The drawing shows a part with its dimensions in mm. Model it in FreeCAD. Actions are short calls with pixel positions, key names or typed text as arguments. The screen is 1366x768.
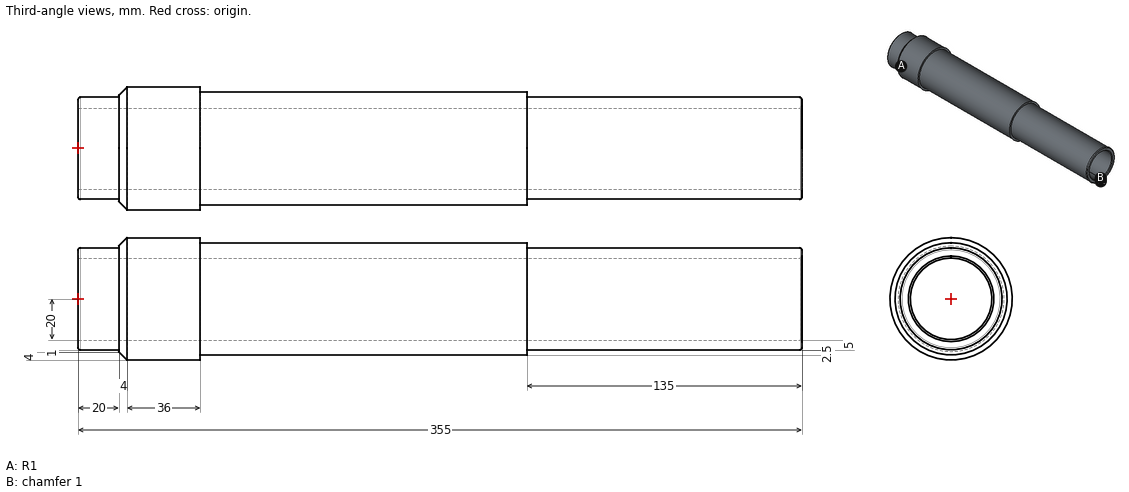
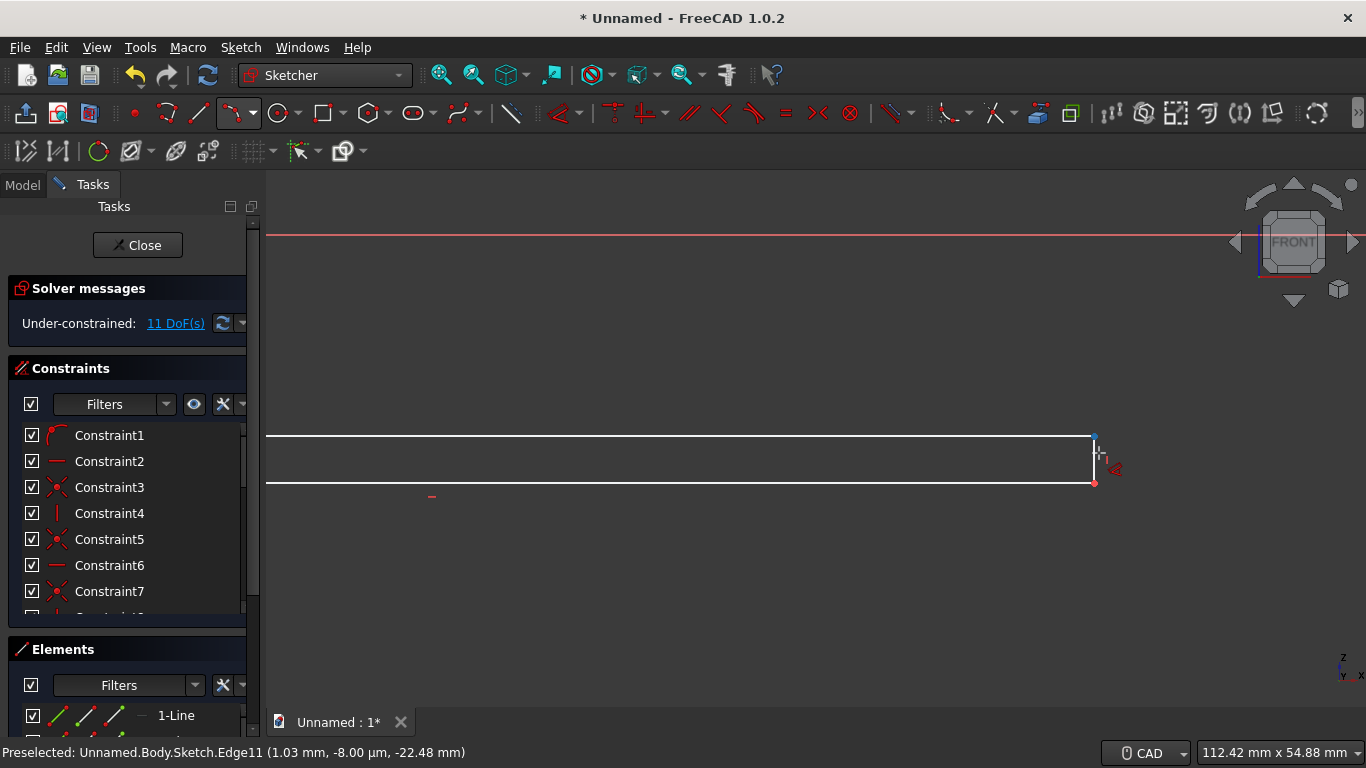
click(1094, 450)
click(1128, 460)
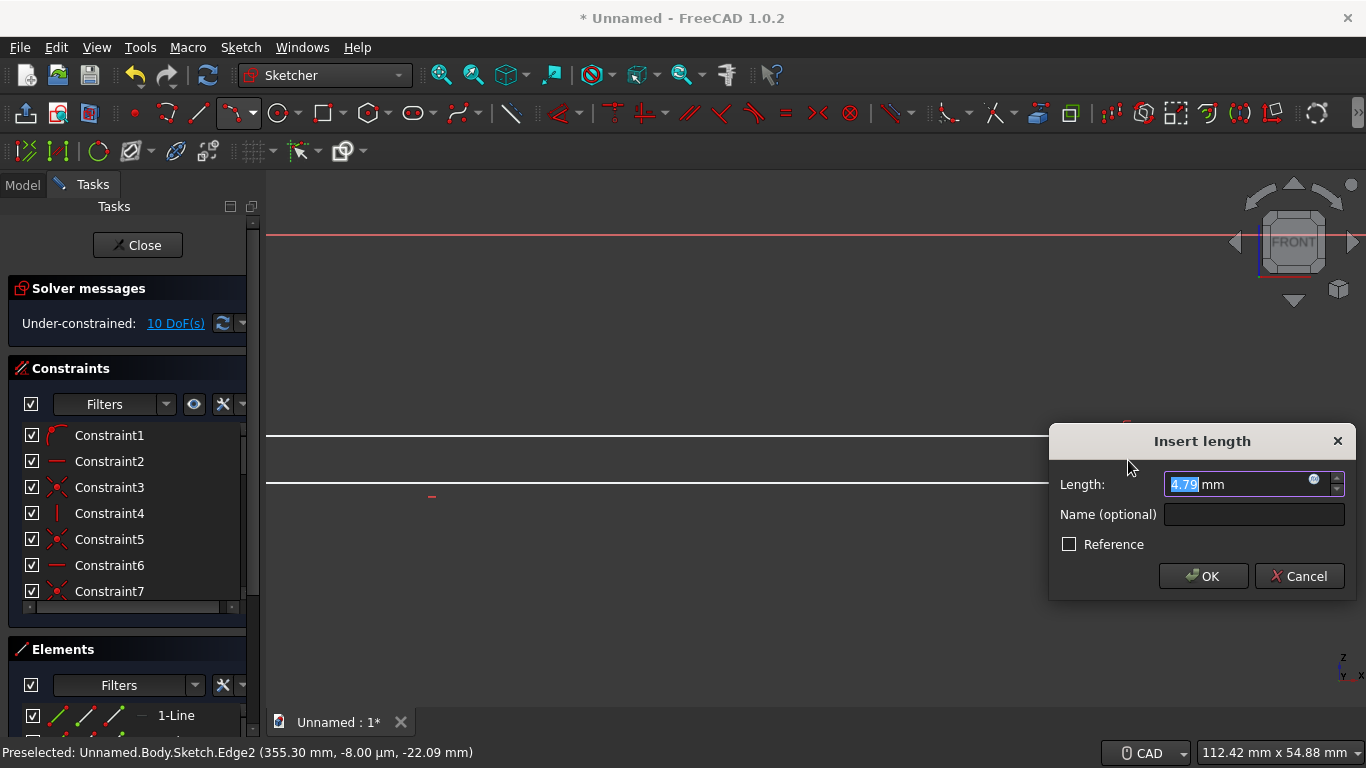
text(5)
key(Return)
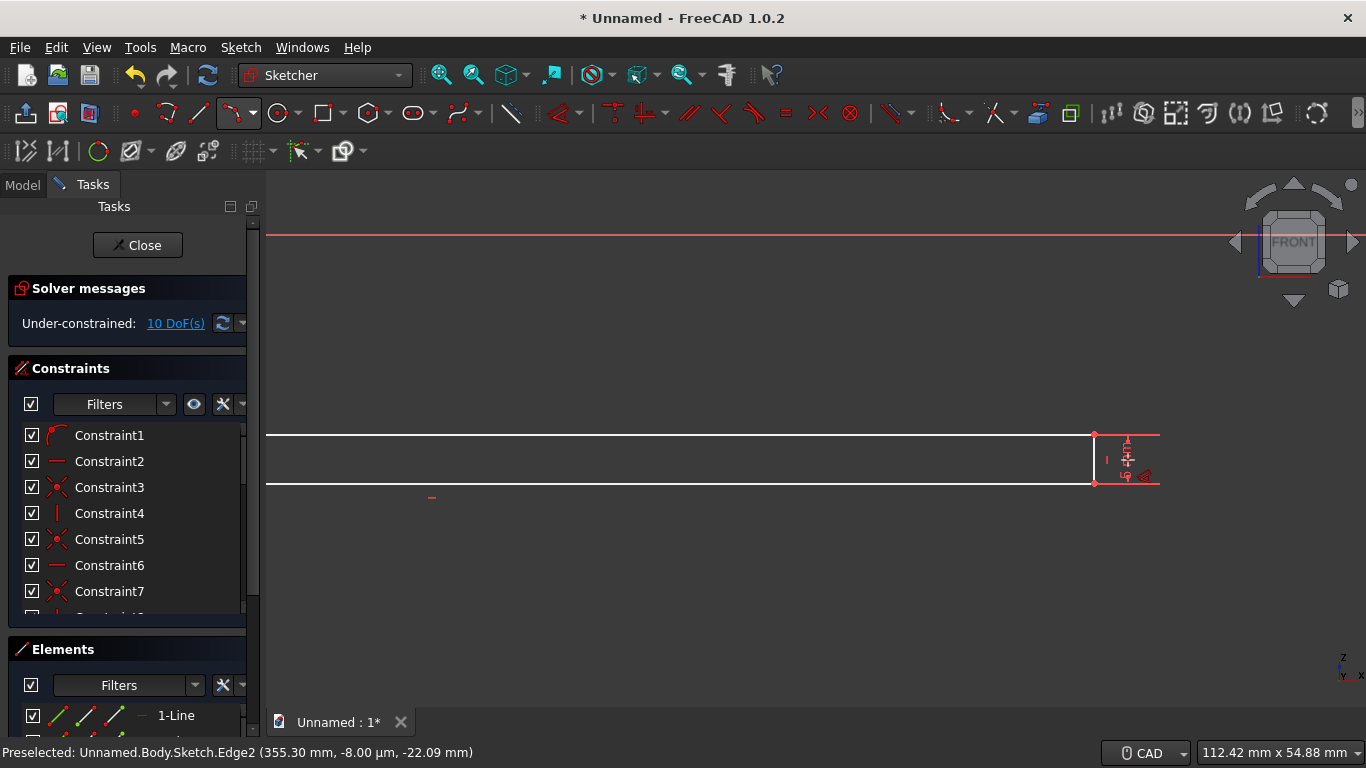
scroll(1100, 453, down, 8)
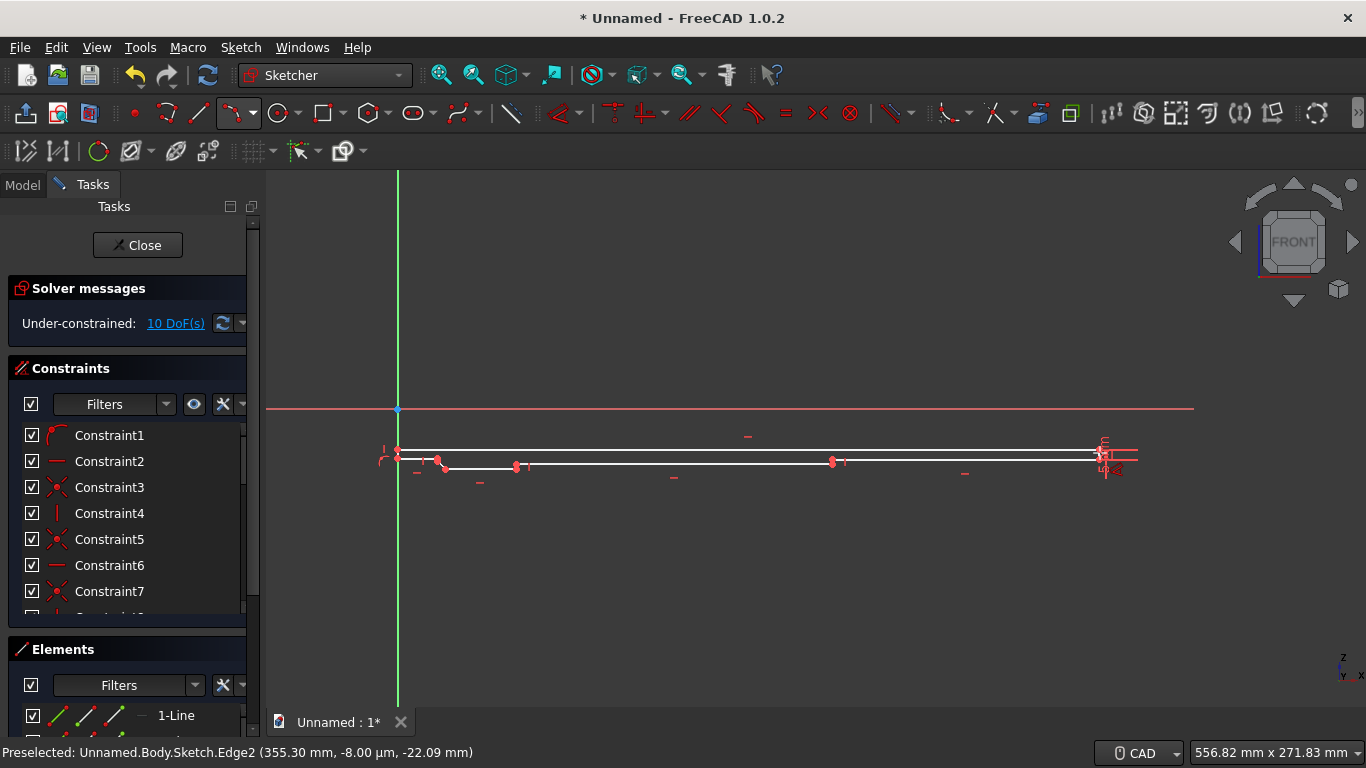
scroll(437, 460, up, 16)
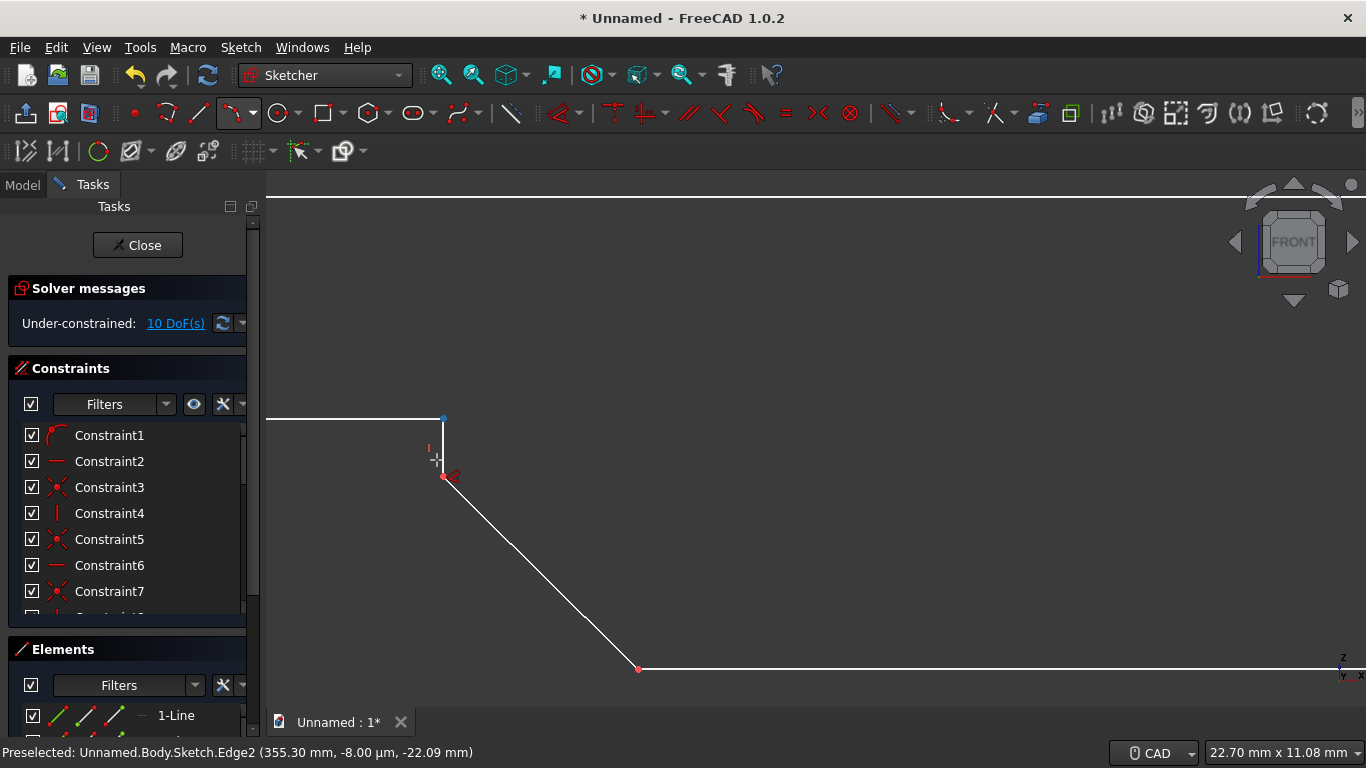
click(443, 448)
click(409, 448)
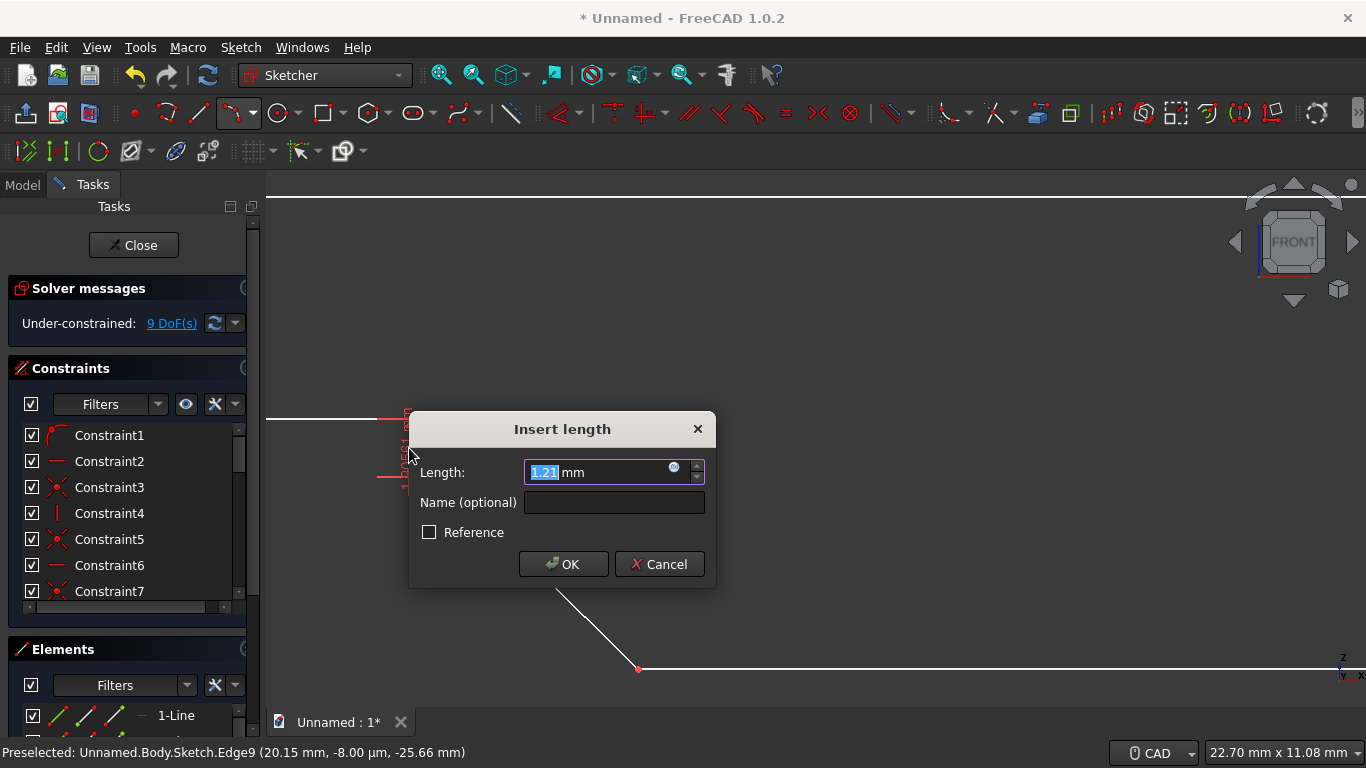
text(1)
key(Return)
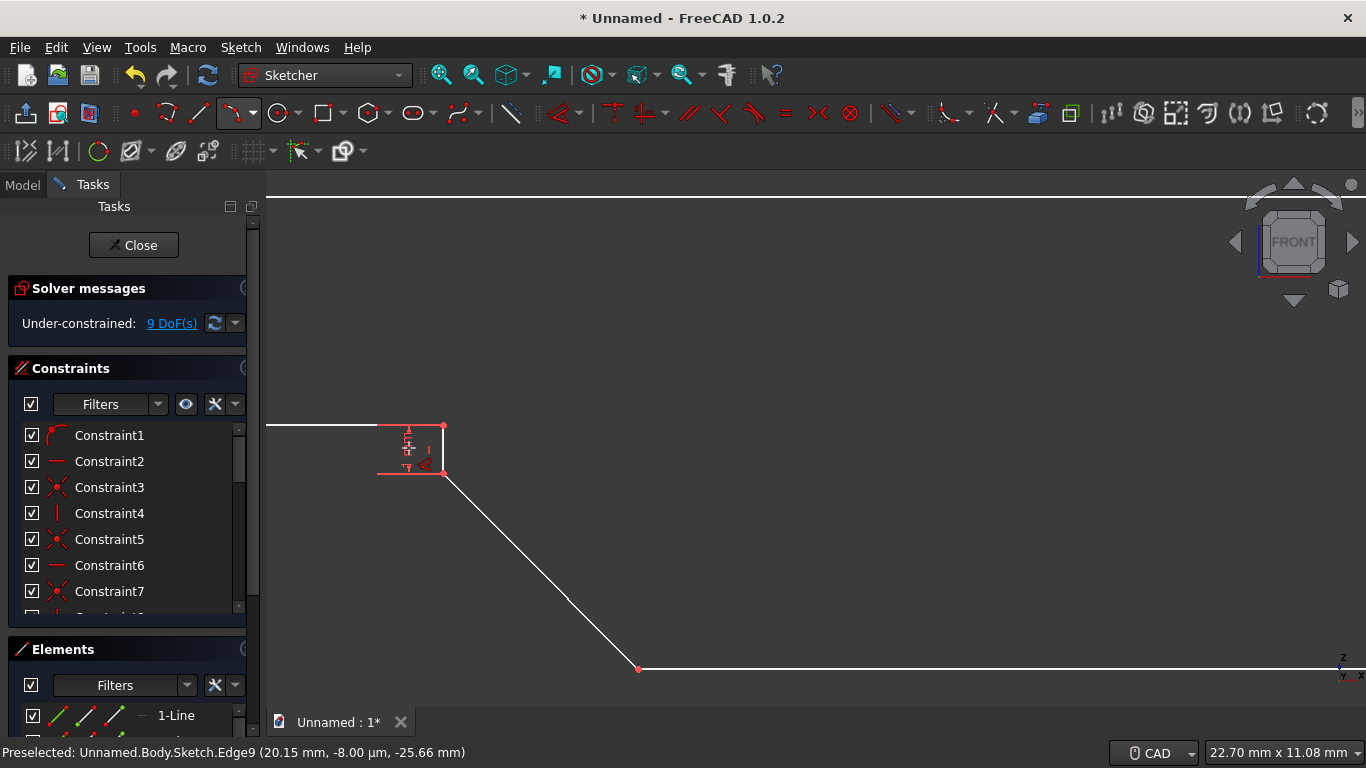
scroll(364, 465, down, 15)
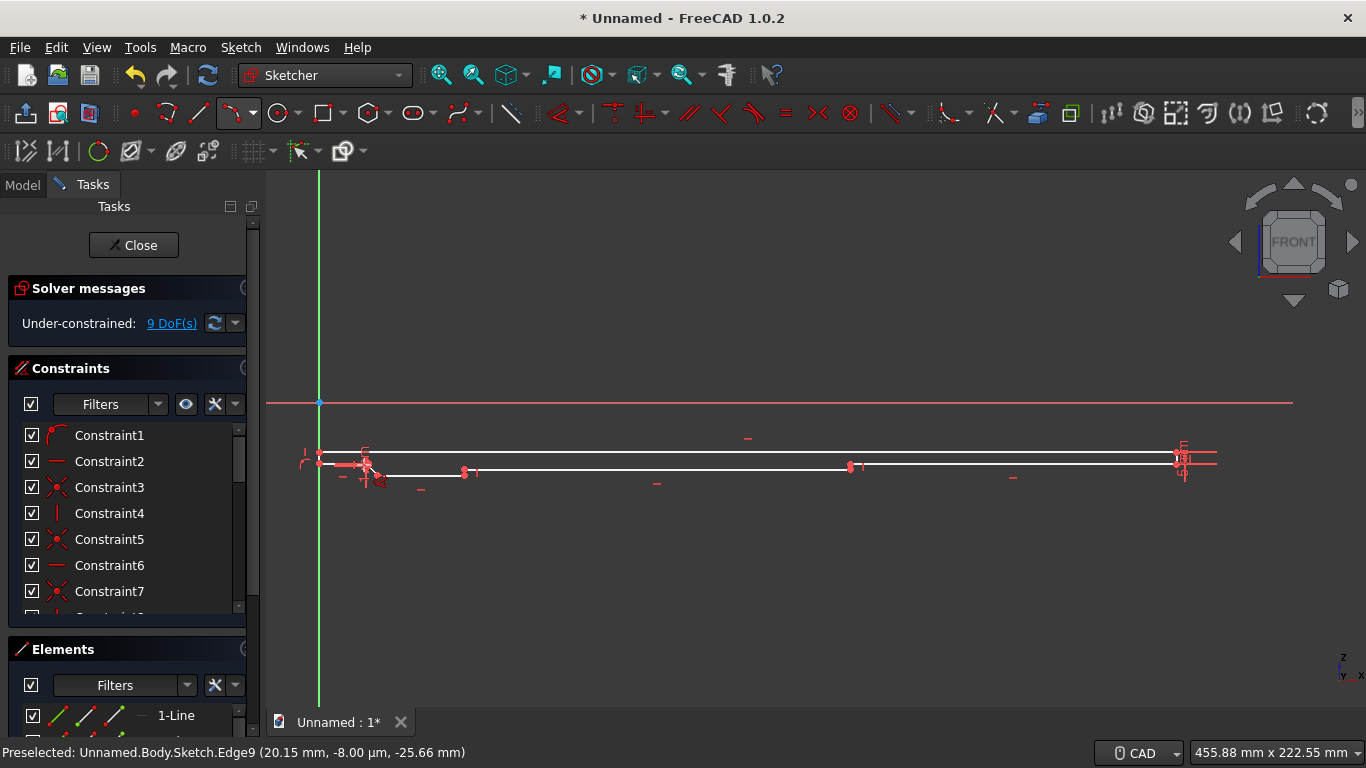
scroll(319, 460, up, 7)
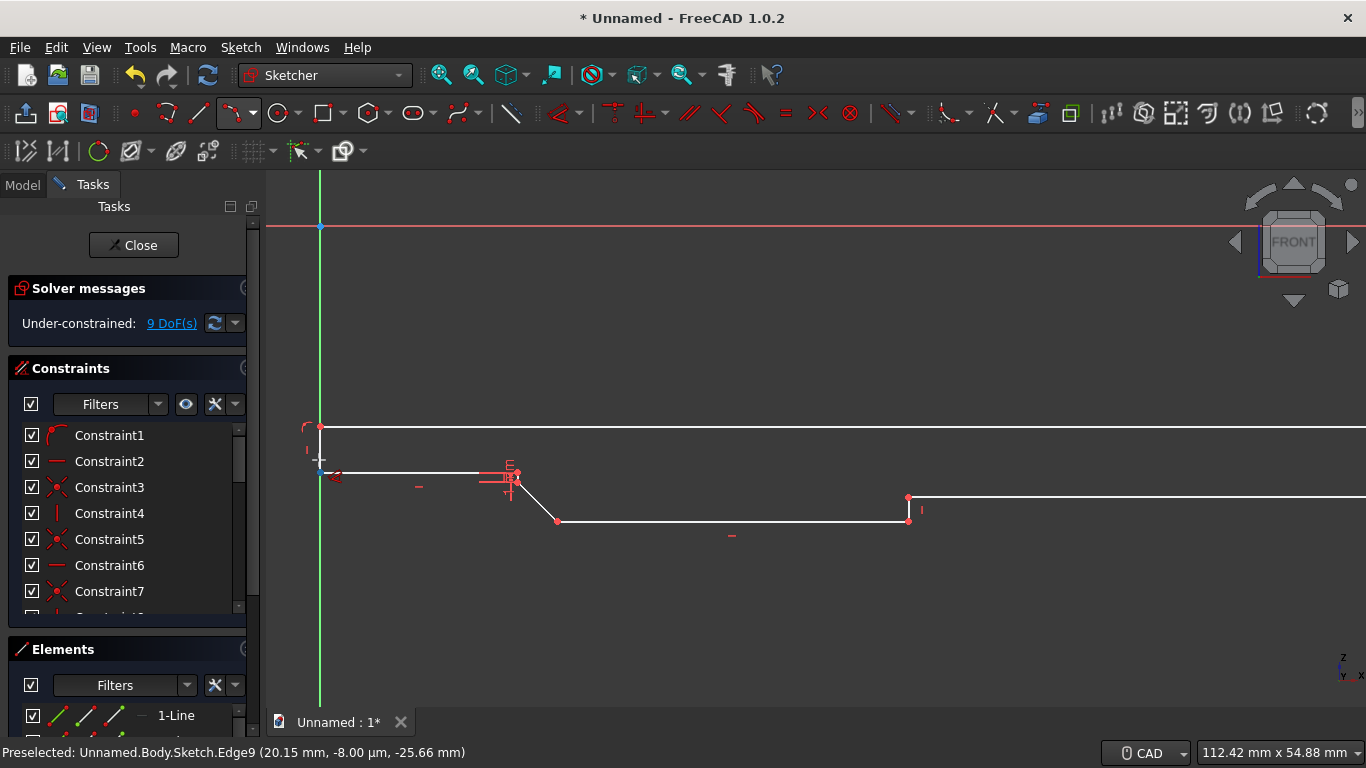
click(320, 459)
click(354, 450)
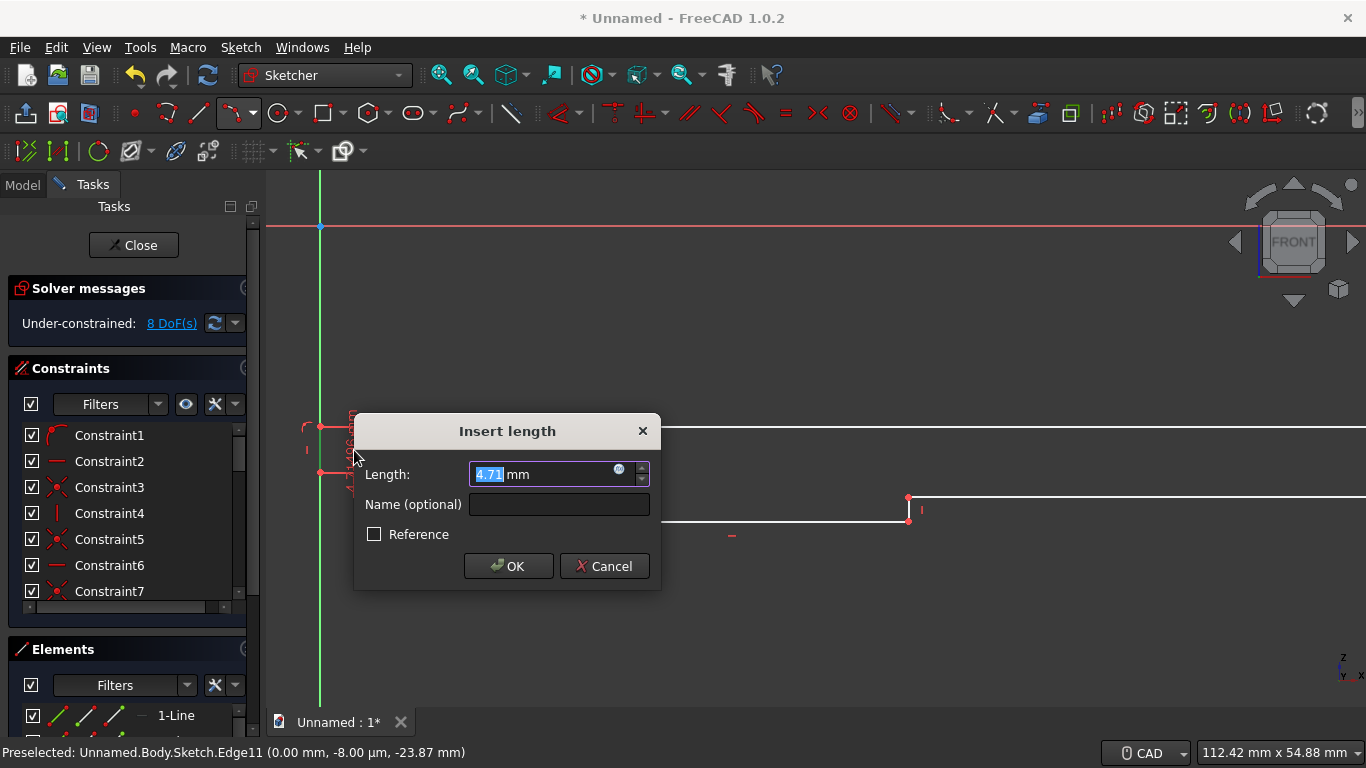
text(5)
key(Return)